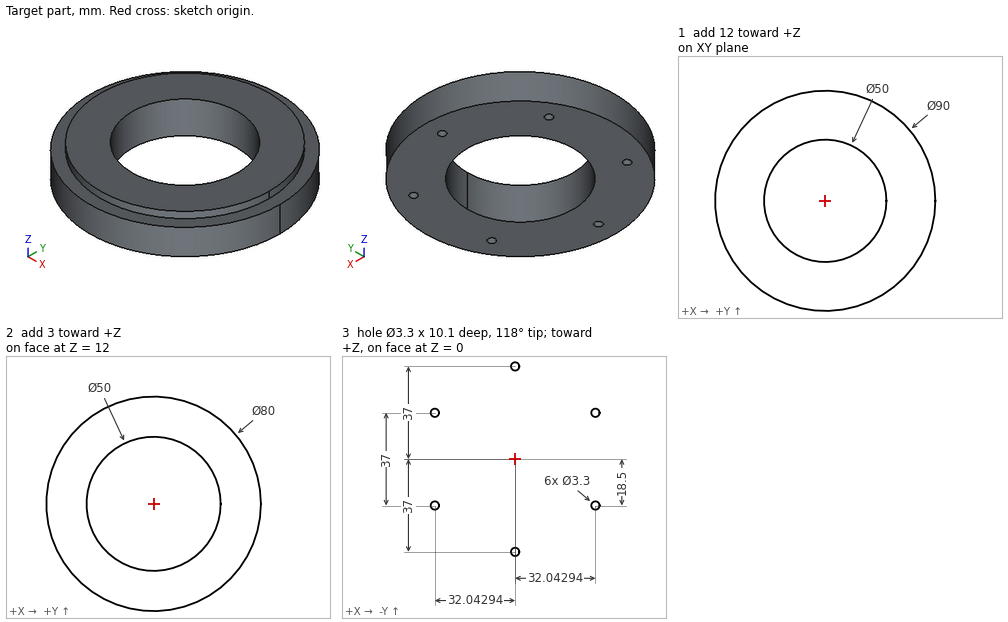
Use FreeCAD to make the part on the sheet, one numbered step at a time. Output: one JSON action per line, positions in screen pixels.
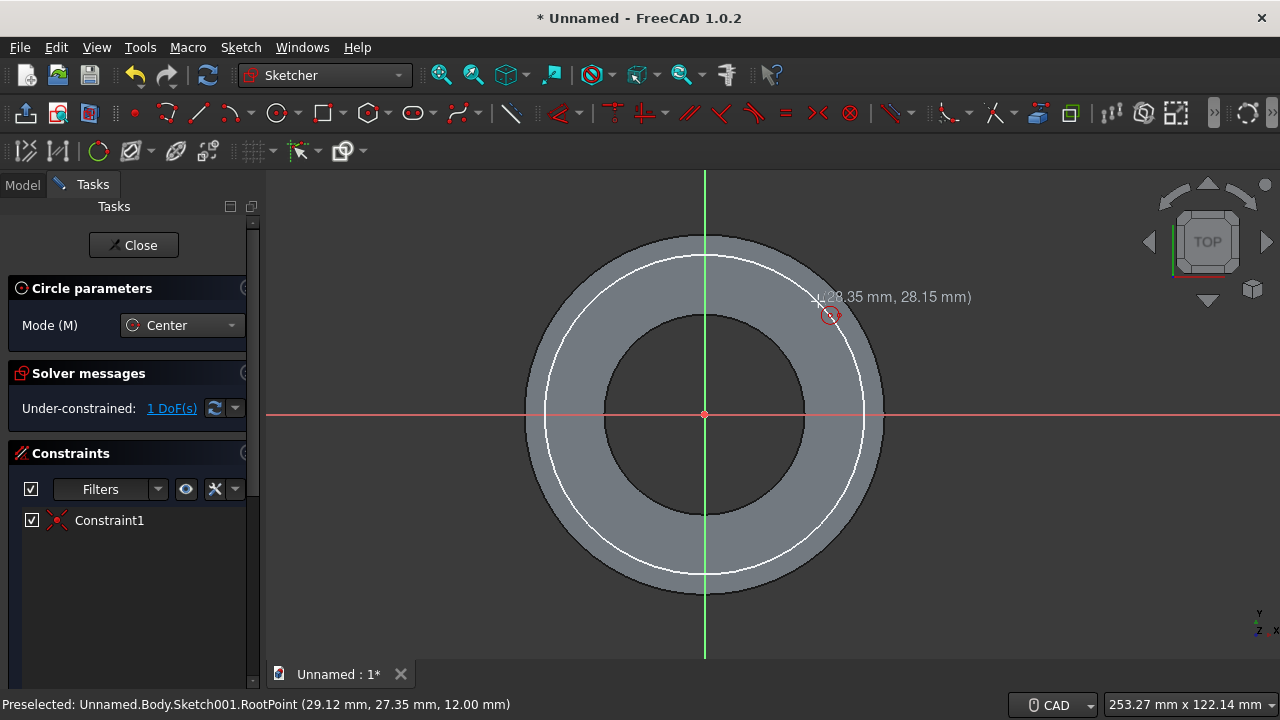
{"action": "left_click", "coordinate": [705, 415]}
{"action": "left_click", "coordinate": [775, 344]}
{"action": "key", "text": "Escape"}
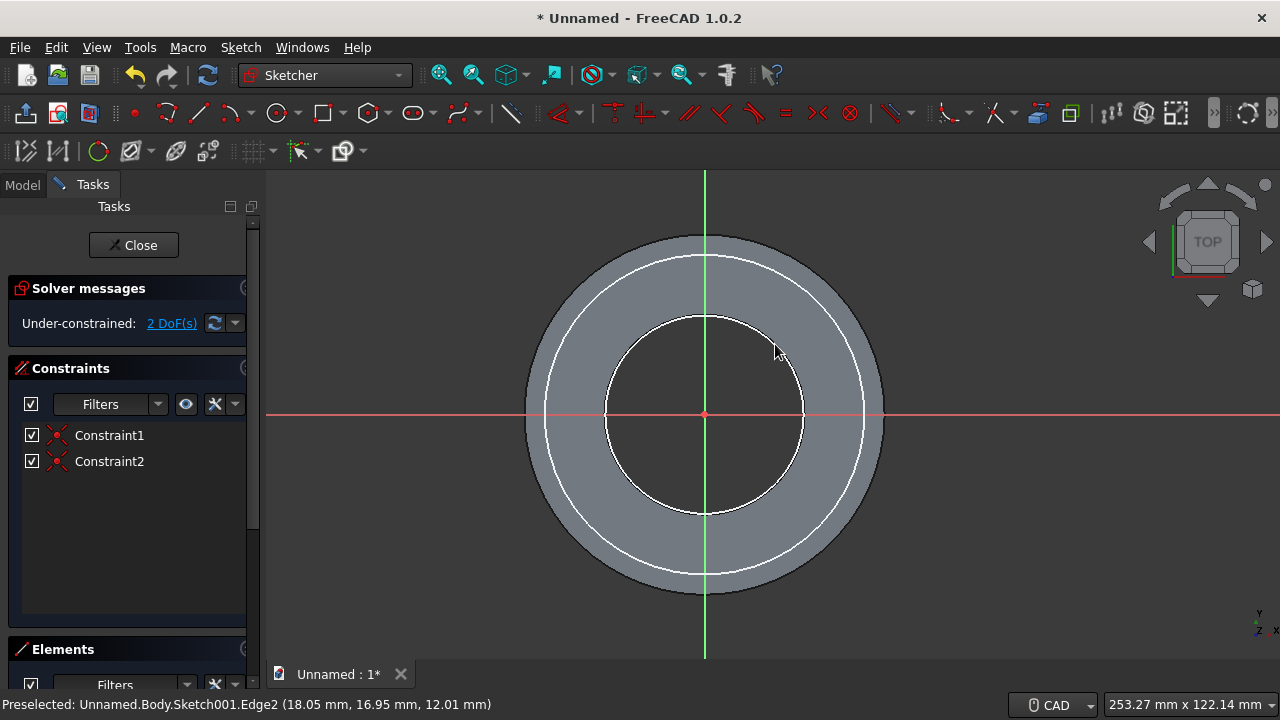
{"action": "left_click", "coordinate": [558, 114]}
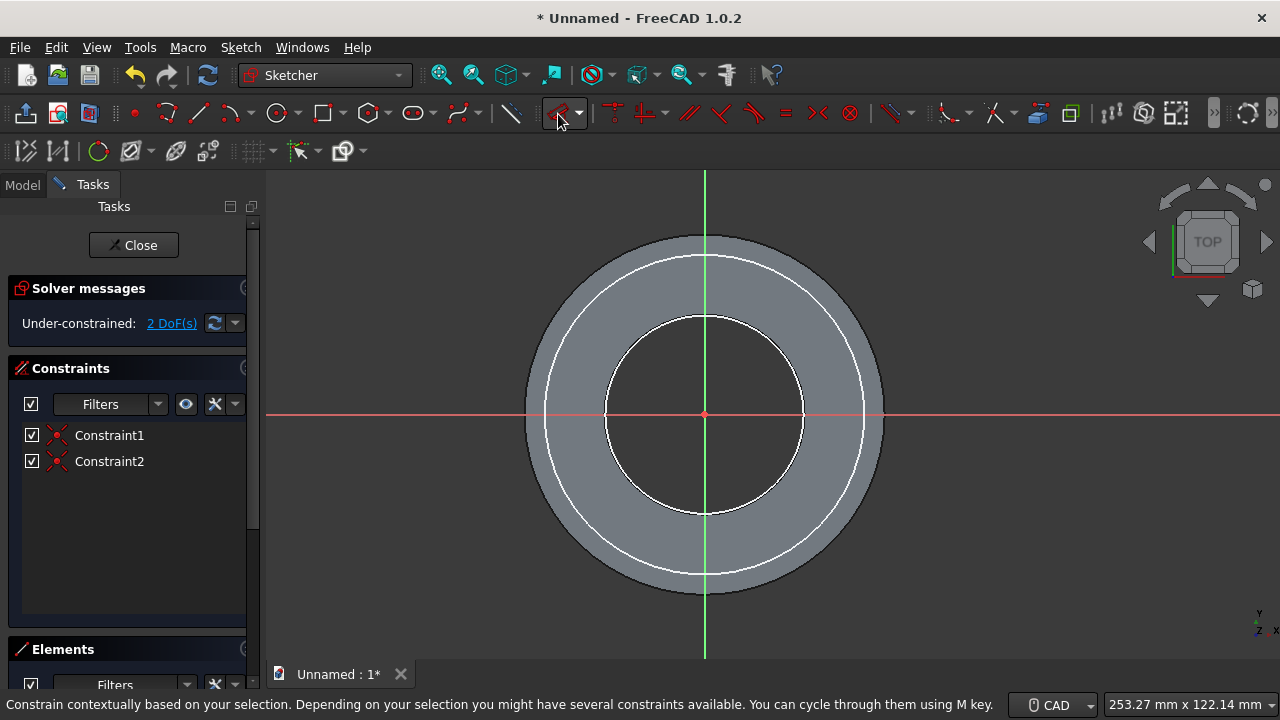
{"action": "left_click", "coordinate": [817, 301]}
{"action": "left_click", "coordinate": [840, 278]}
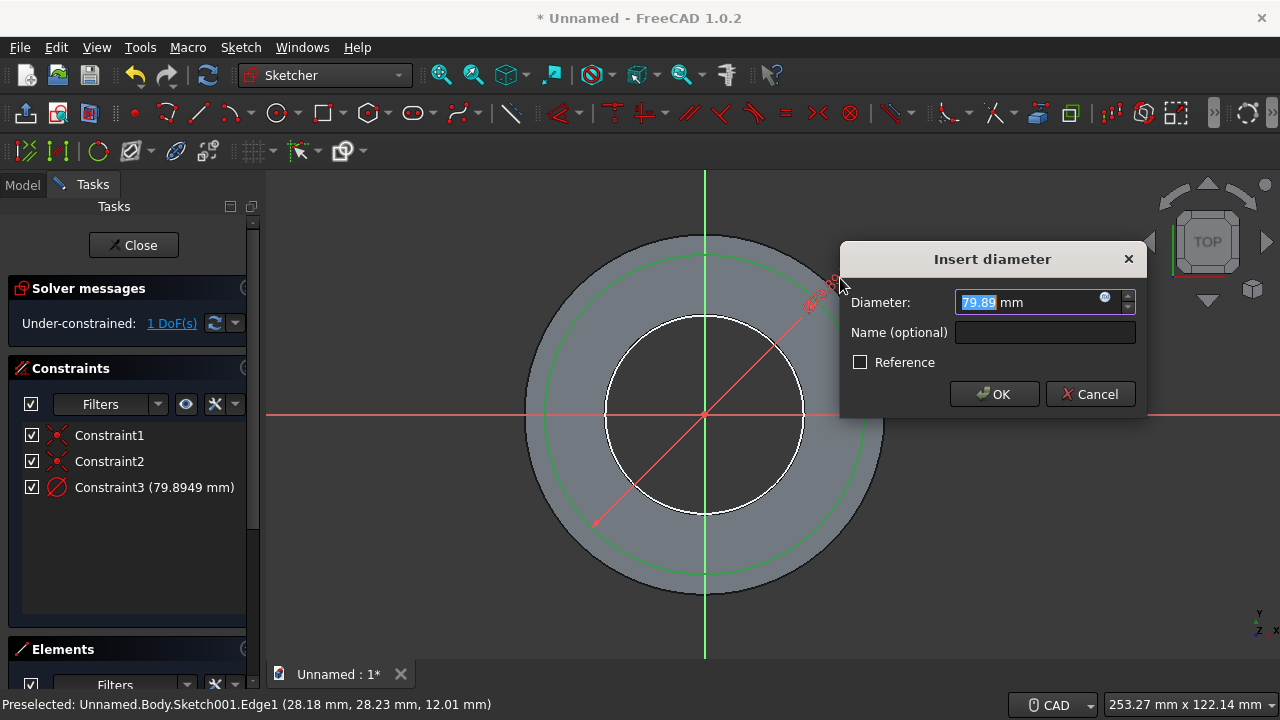
{"action": "type", "text": "80"}
{"action": "key", "text": "Return"}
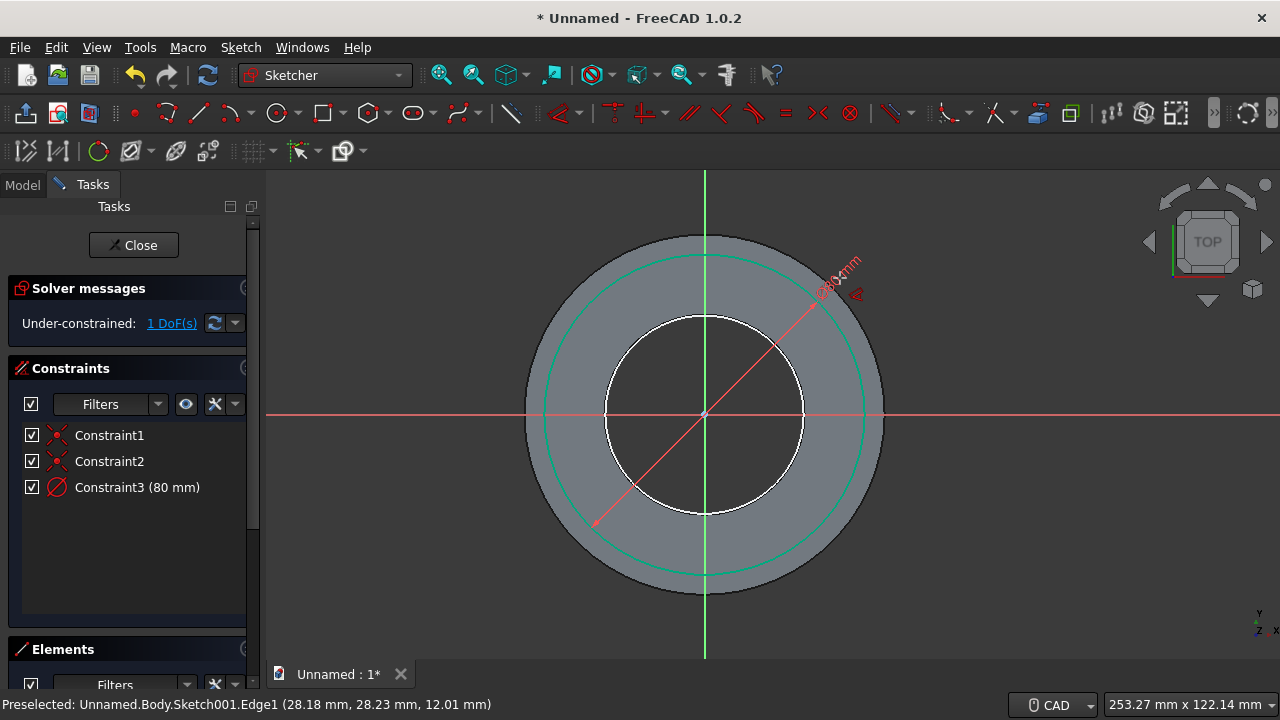
{"action": "left_click", "coordinate": [774, 344]}
{"action": "left_click", "coordinate": [796, 321]}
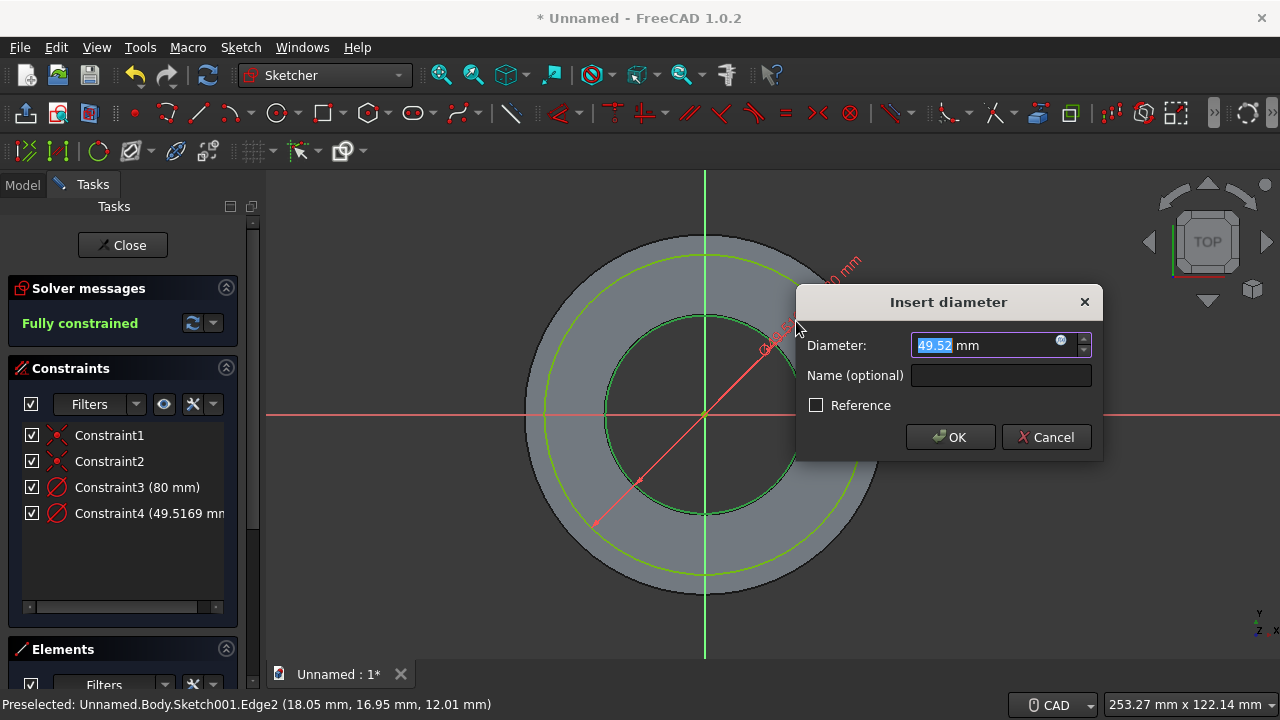
{"action": "type", "text": "50"}
{"action": "key", "text": "Return"}
{"action": "key", "text": "Escape"}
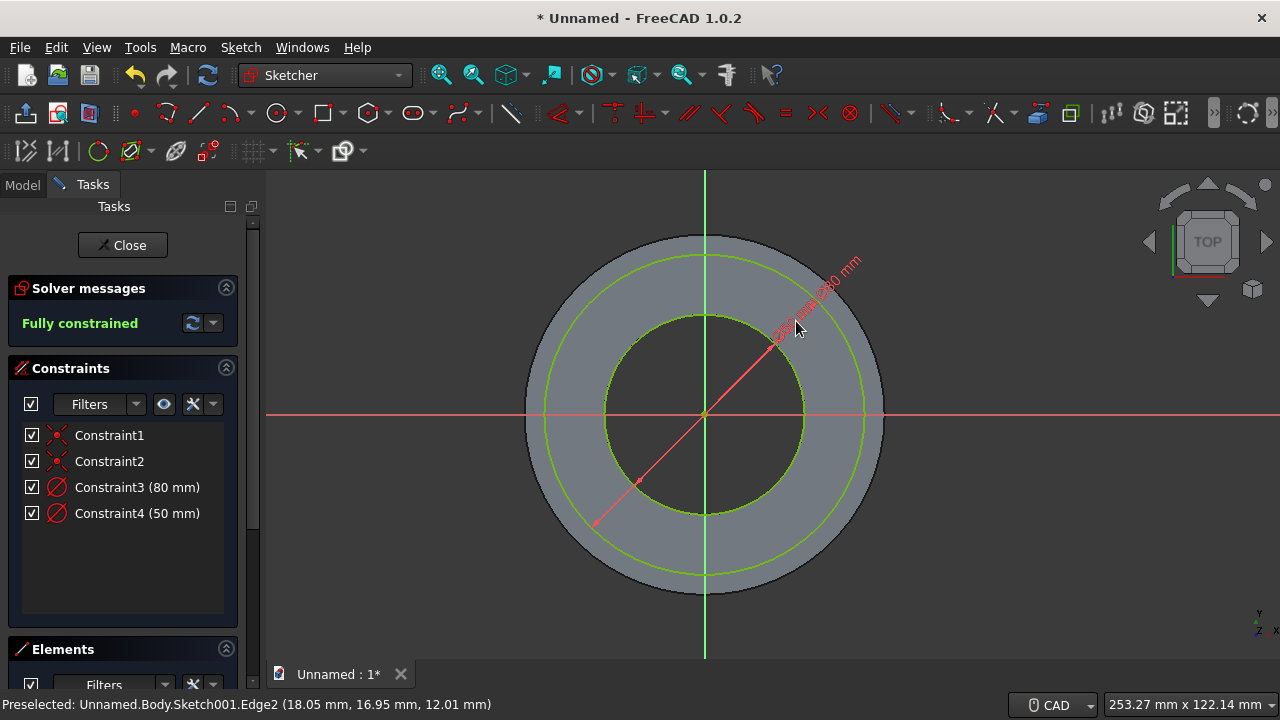
{"action": "left_click", "coordinate": [123, 245]}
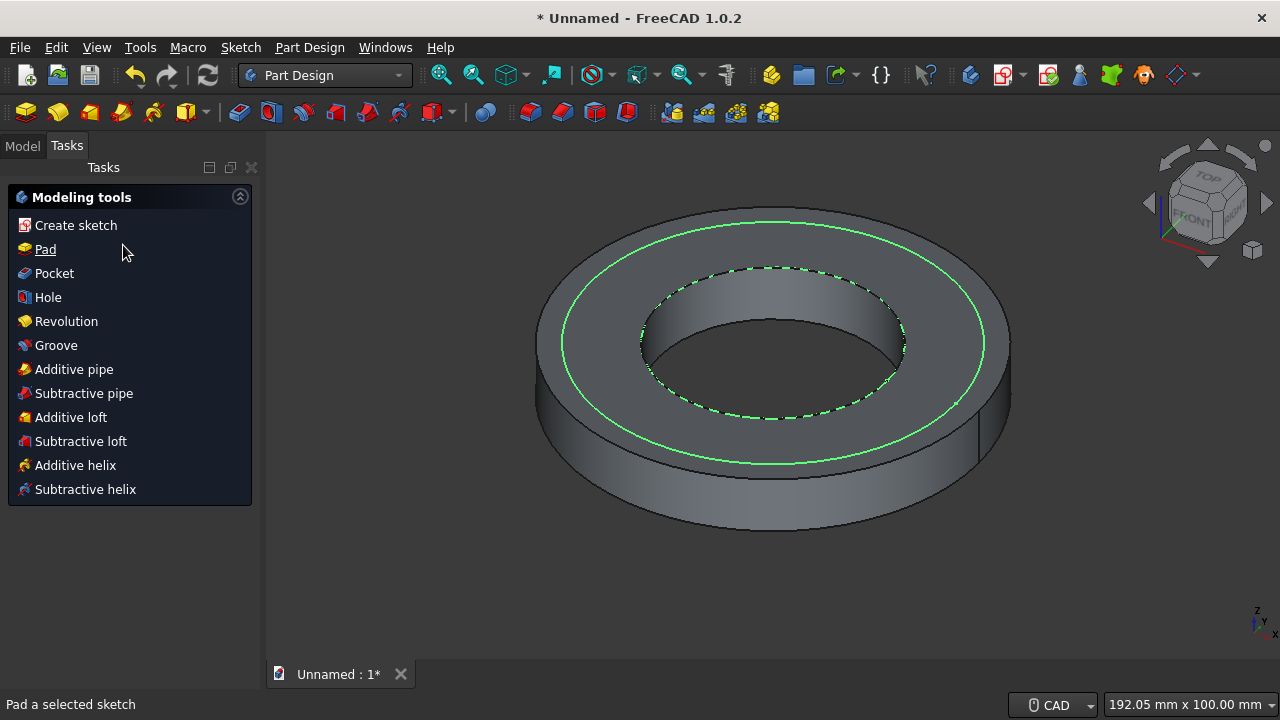
{"action": "left_click", "coordinate": [26, 112]}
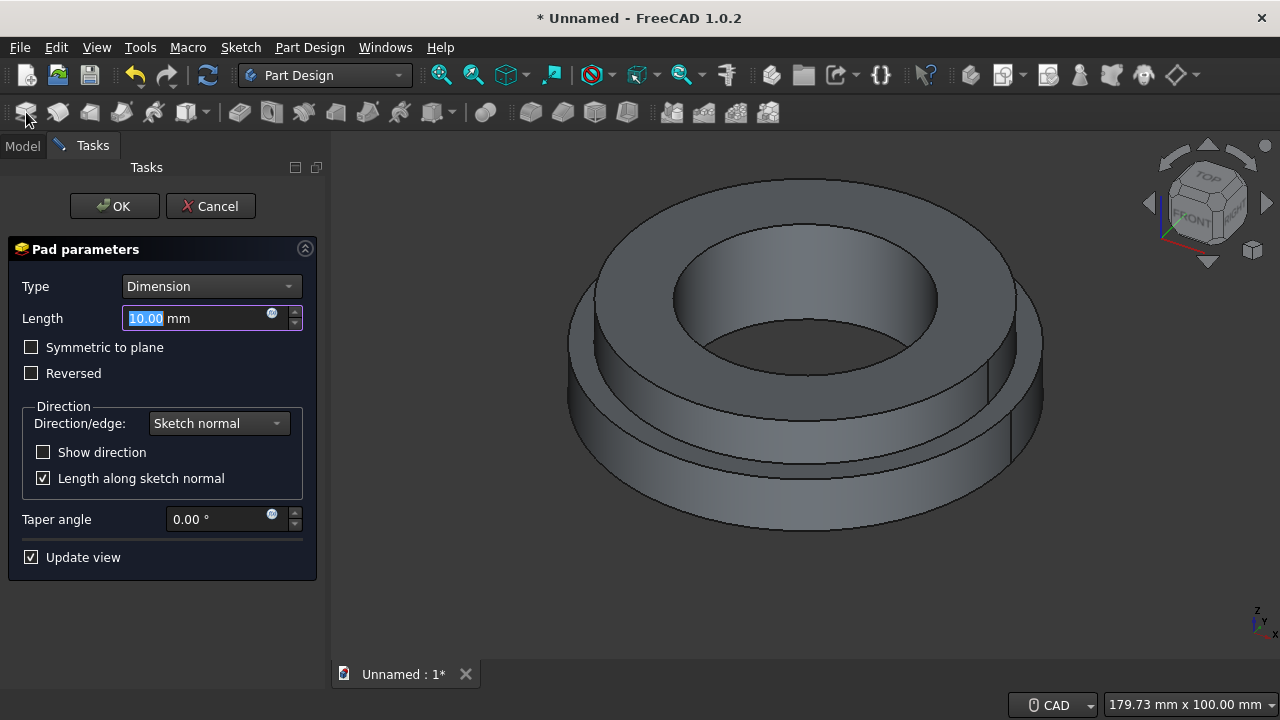
{"action": "type", "text": "3"}
{"action": "key", "text": "Tab"}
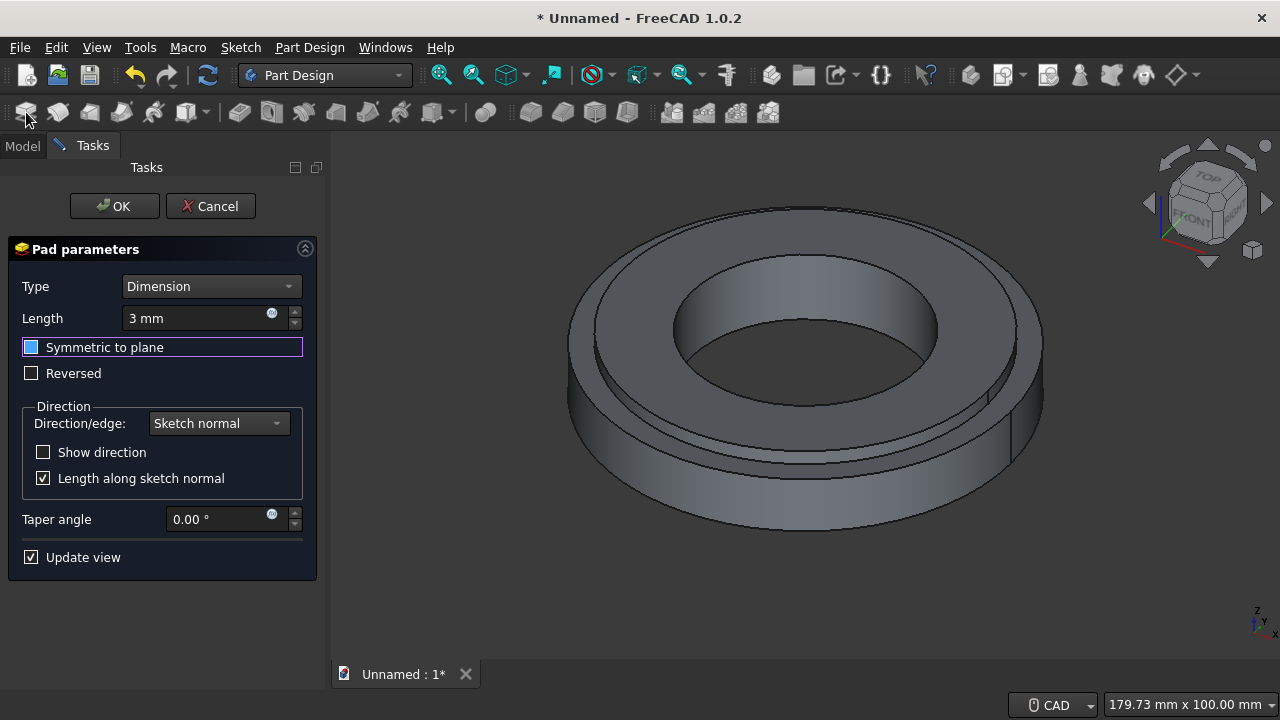
{"action": "left_click", "coordinate": [115, 206]}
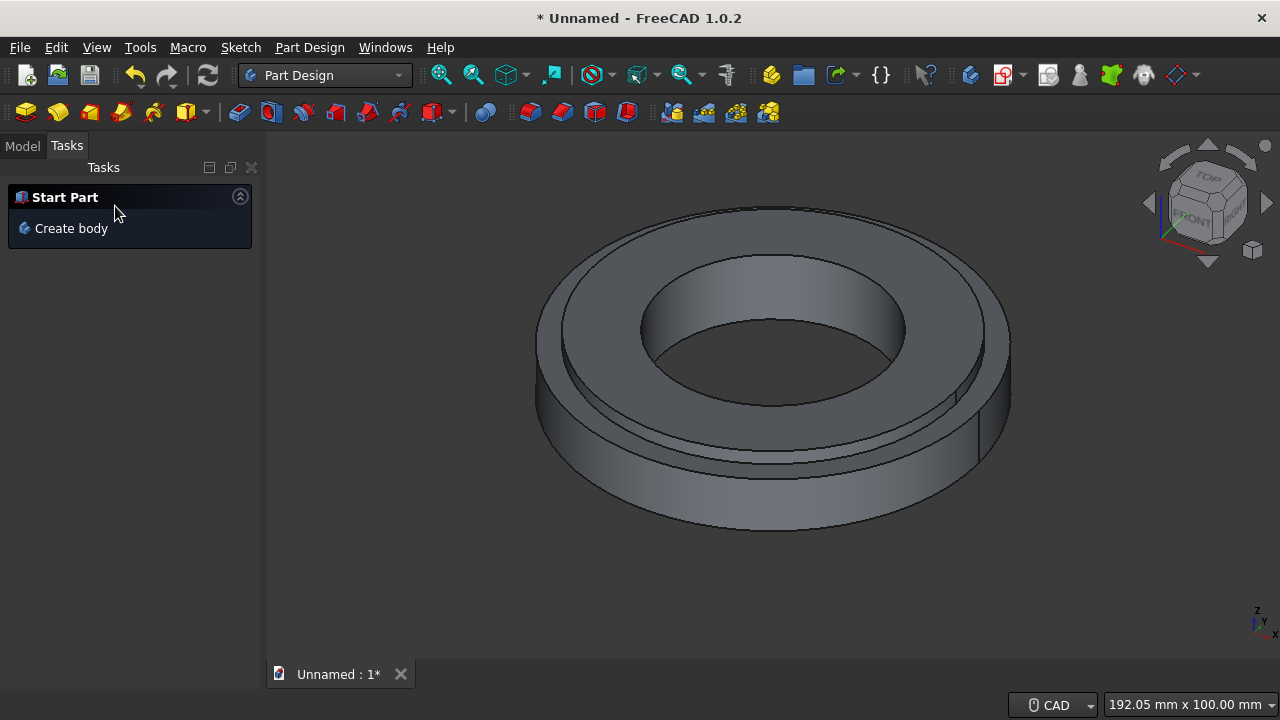
{"action": "key", "text": "5"}